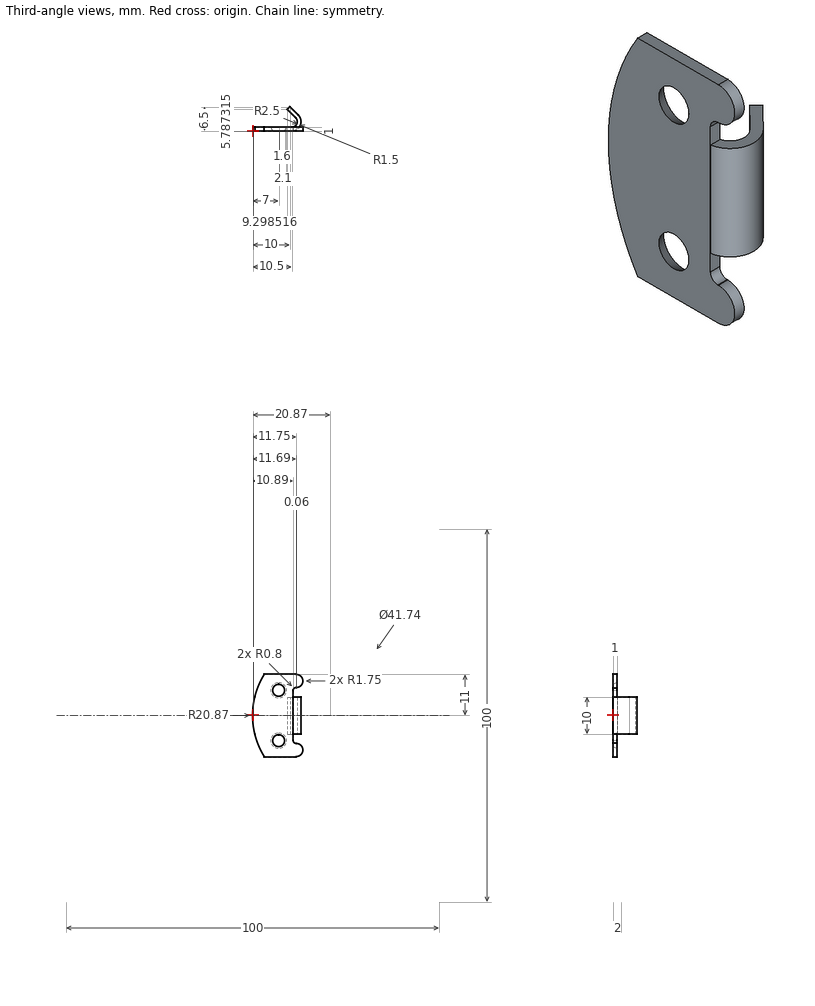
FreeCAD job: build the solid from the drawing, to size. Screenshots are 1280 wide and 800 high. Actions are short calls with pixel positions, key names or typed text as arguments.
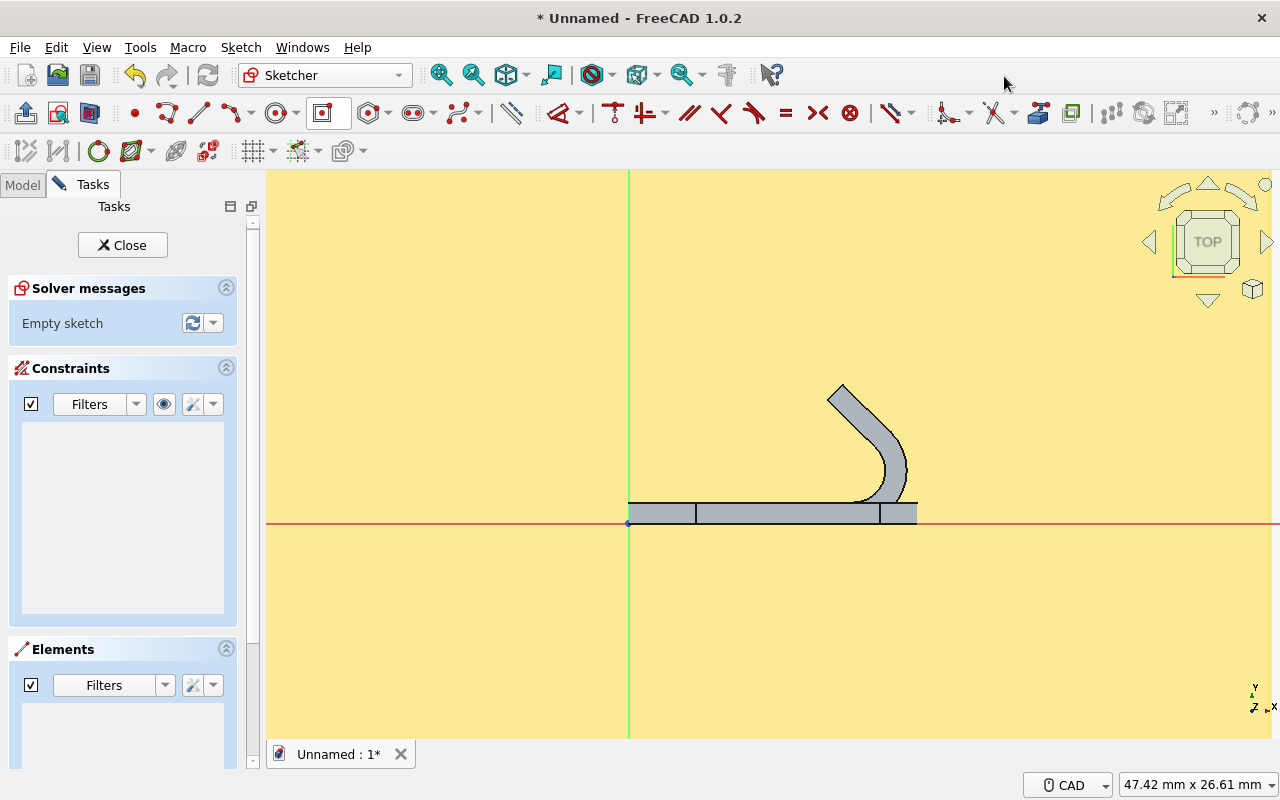
click(90, 114)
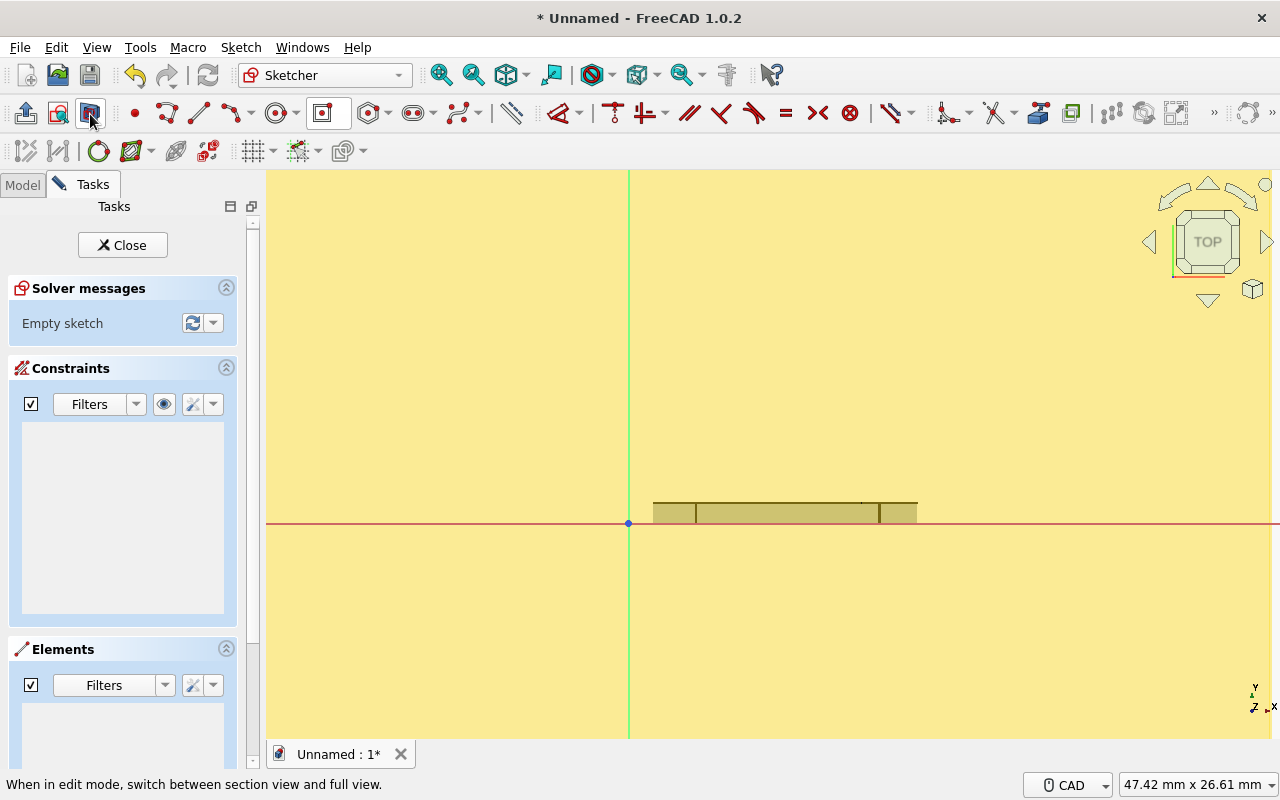
scroll(811, 514, up, 12)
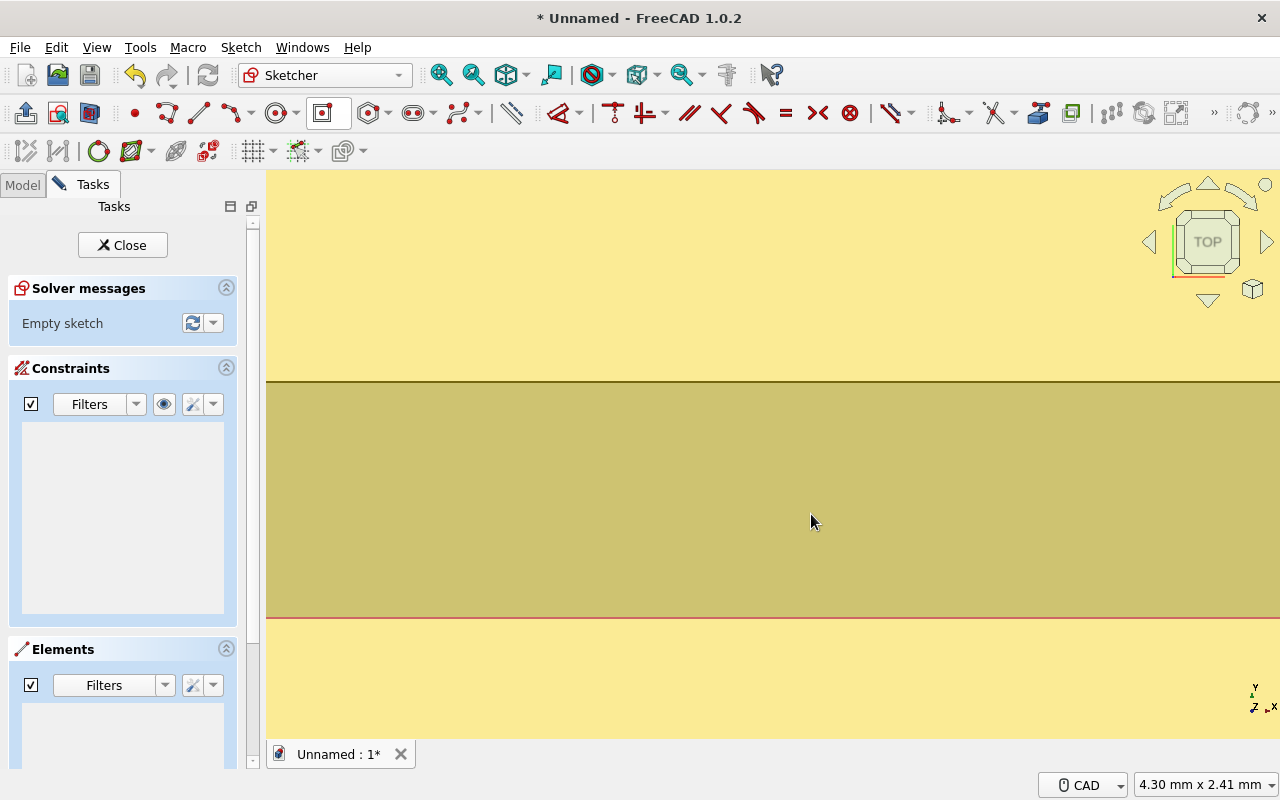
click(168, 114)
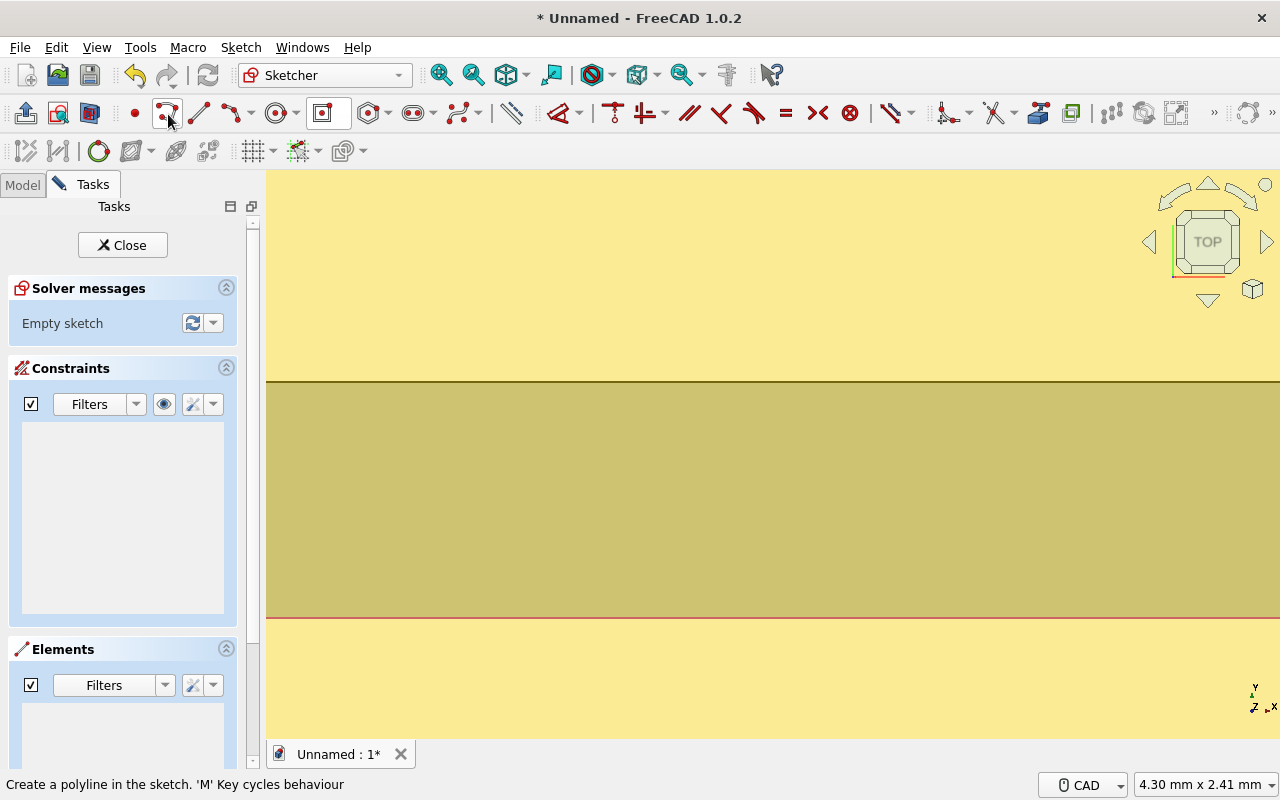
click(447, 618)
click(824, 609)
click(942, 382)
click(447, 382)
click(447, 618)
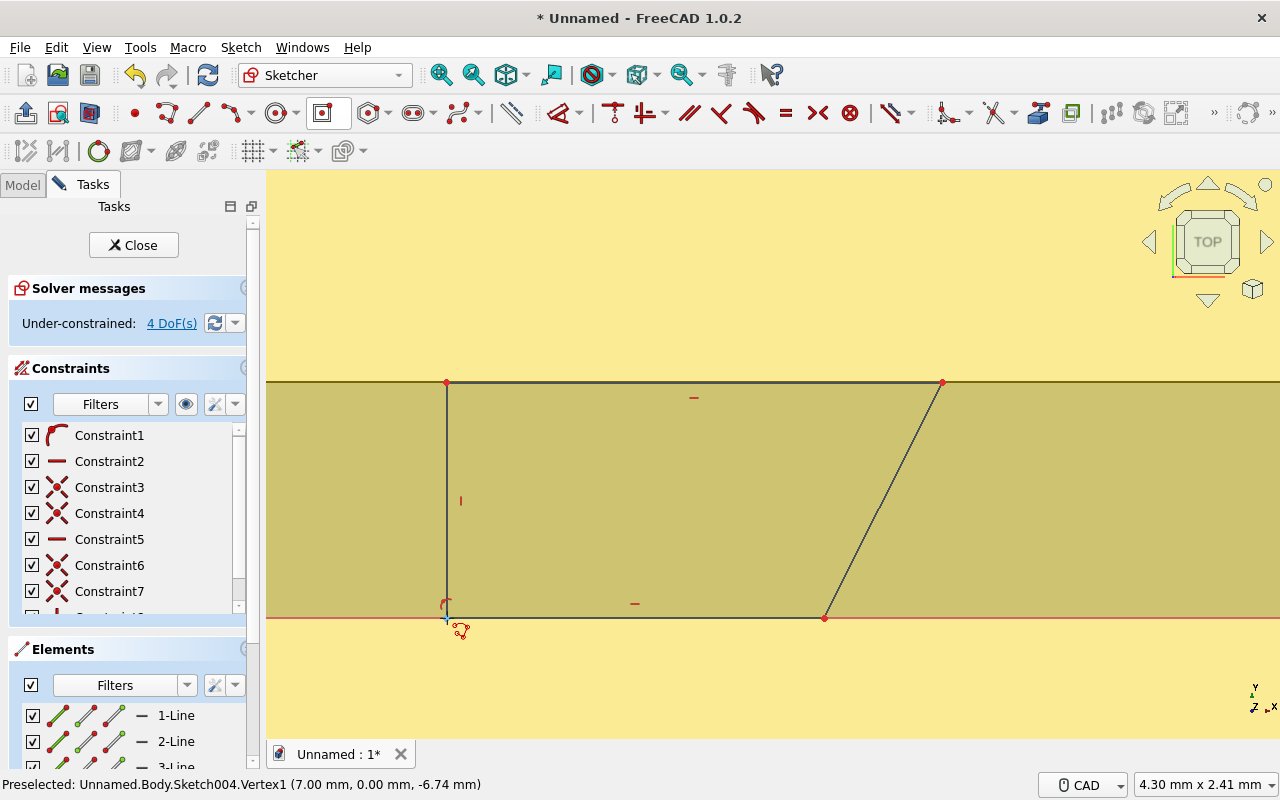
click(200, 114)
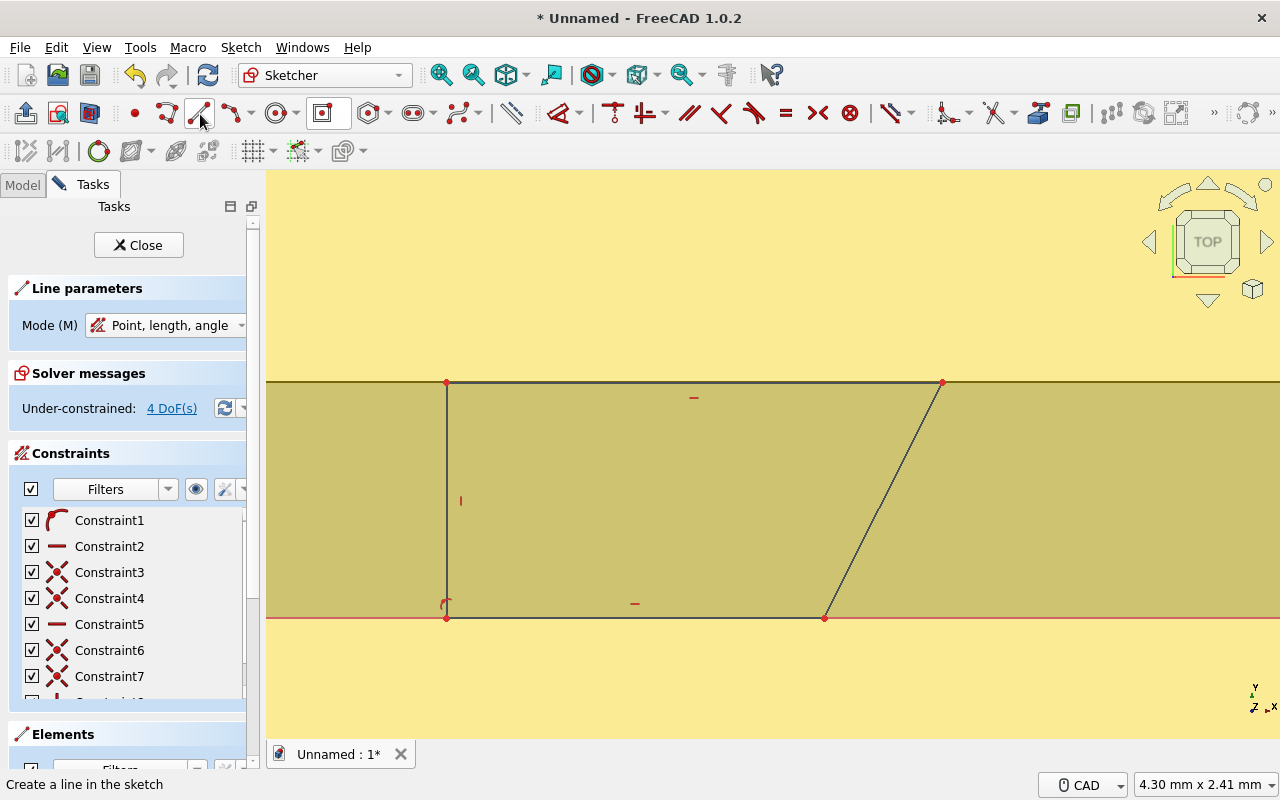
click(447, 359)
click(447, 288)
key(Escape)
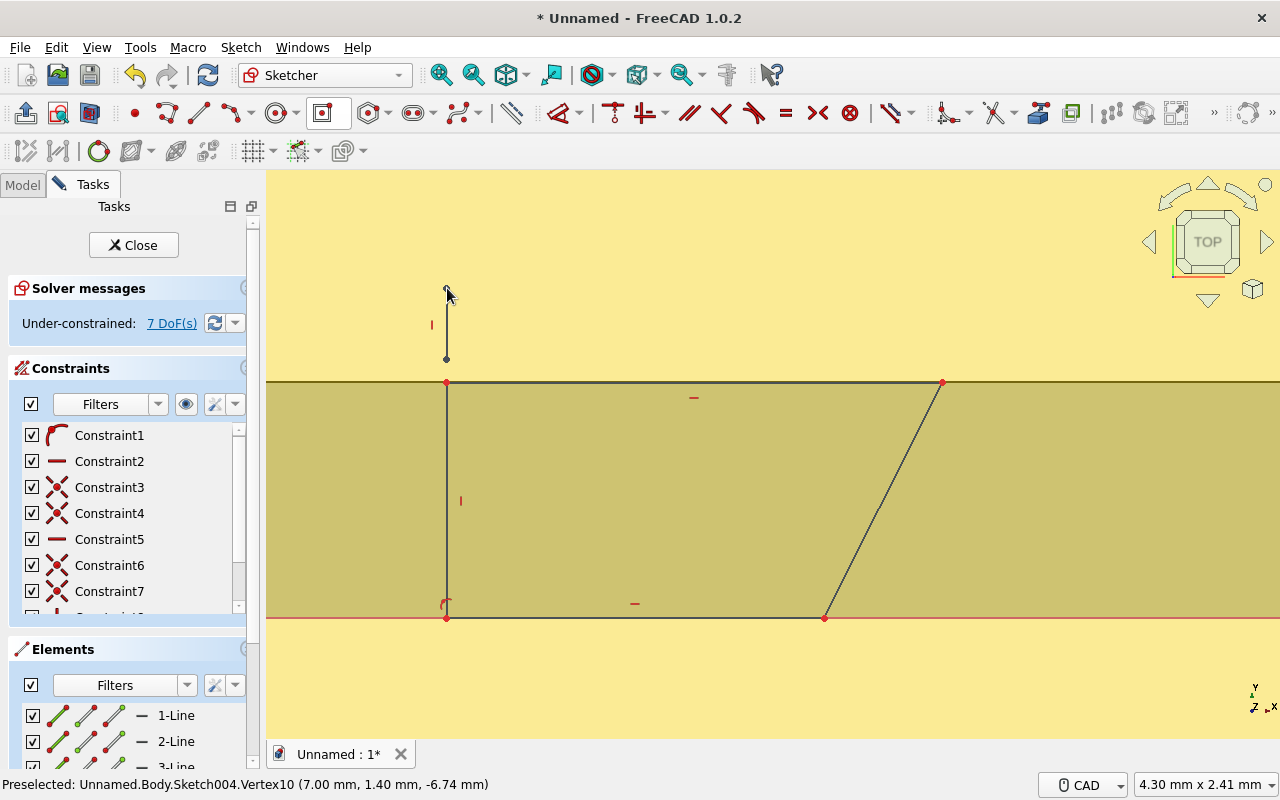
click(447, 339)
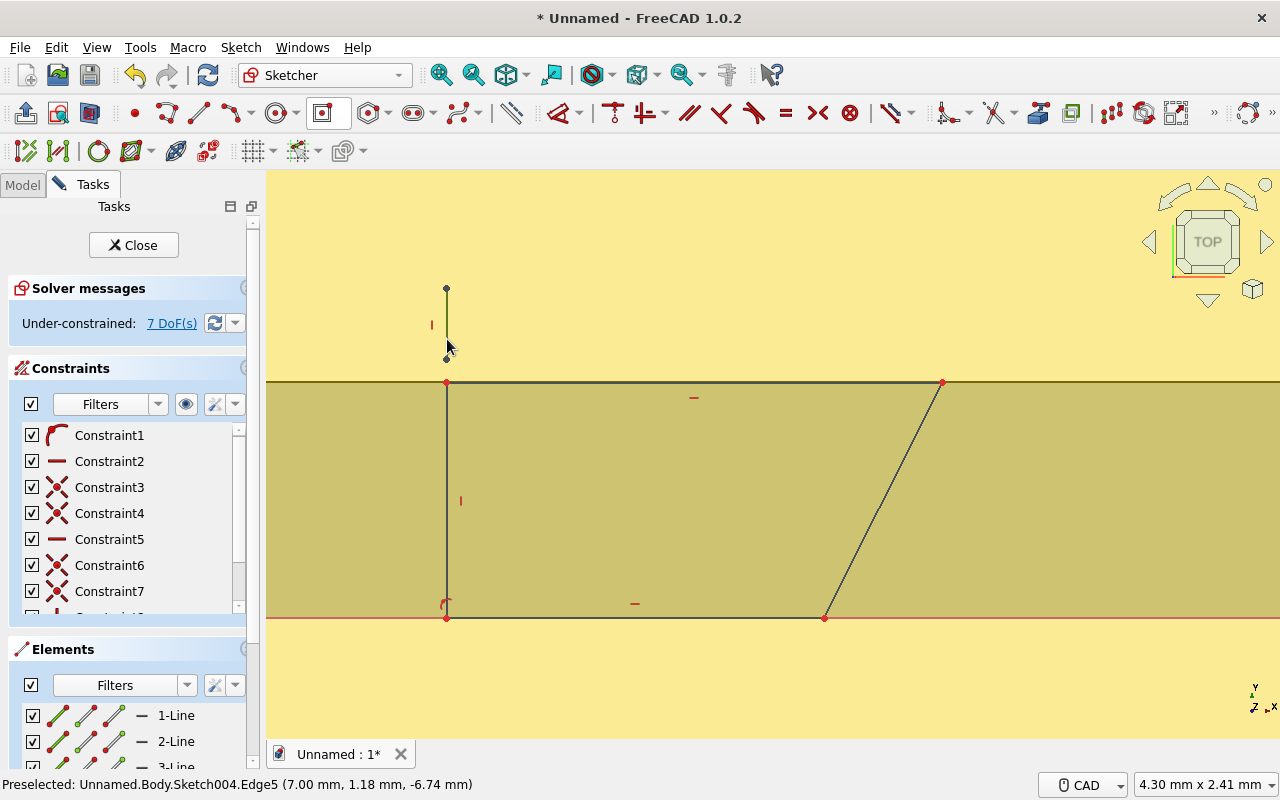
click(512, 114)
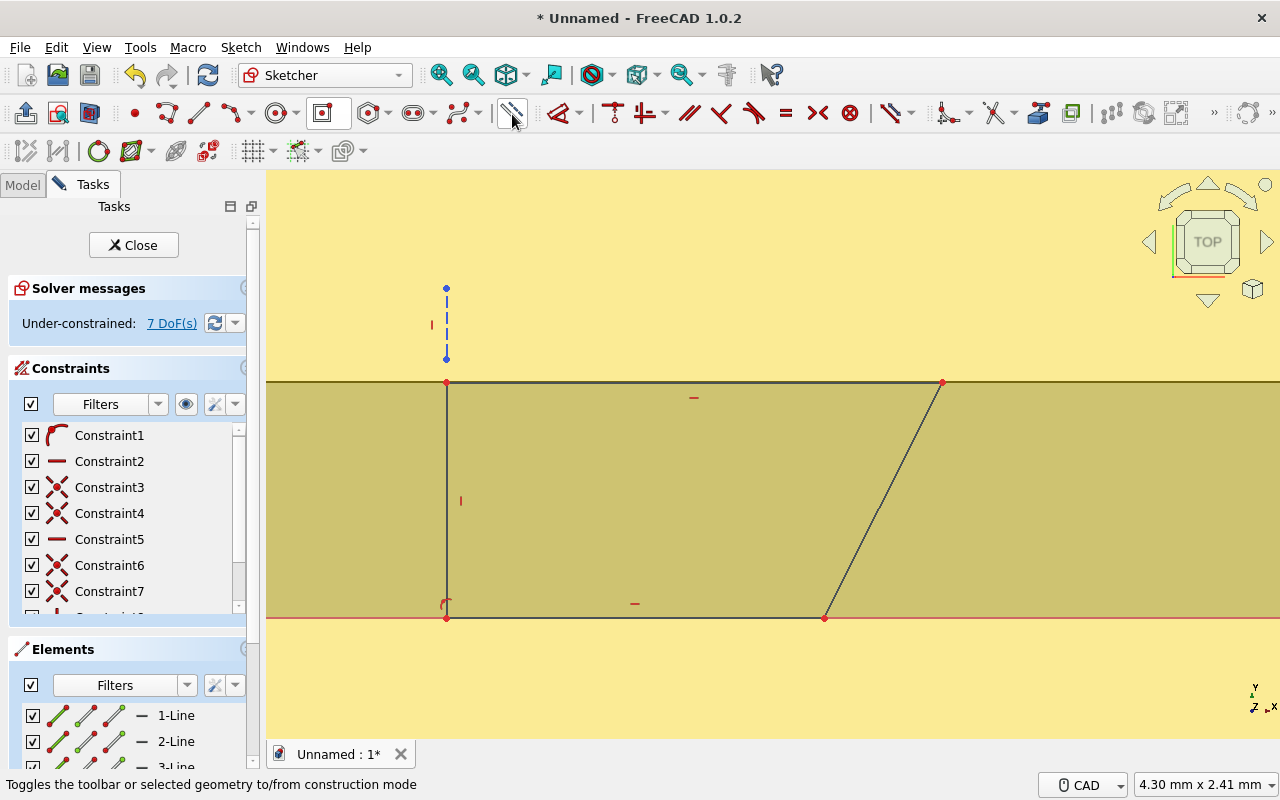
click(558, 114)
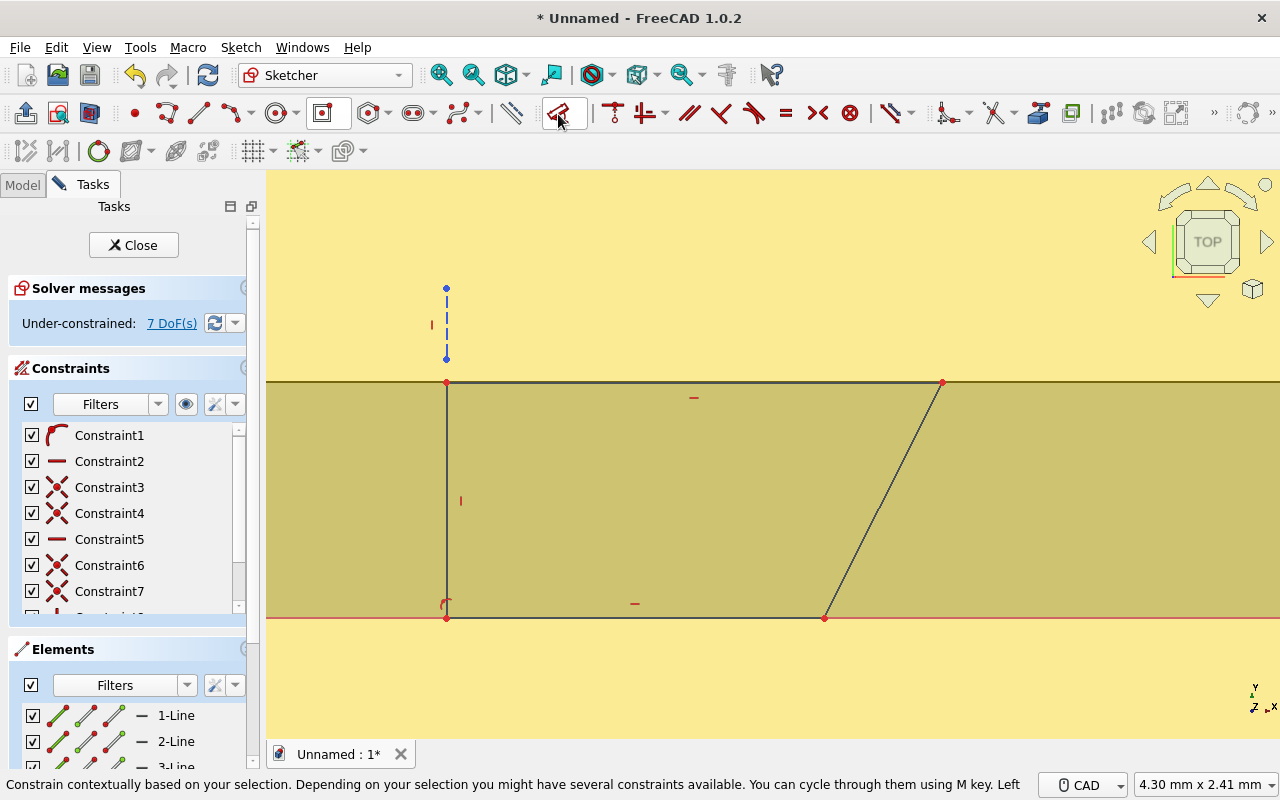
click(447, 454)
click(413, 501)